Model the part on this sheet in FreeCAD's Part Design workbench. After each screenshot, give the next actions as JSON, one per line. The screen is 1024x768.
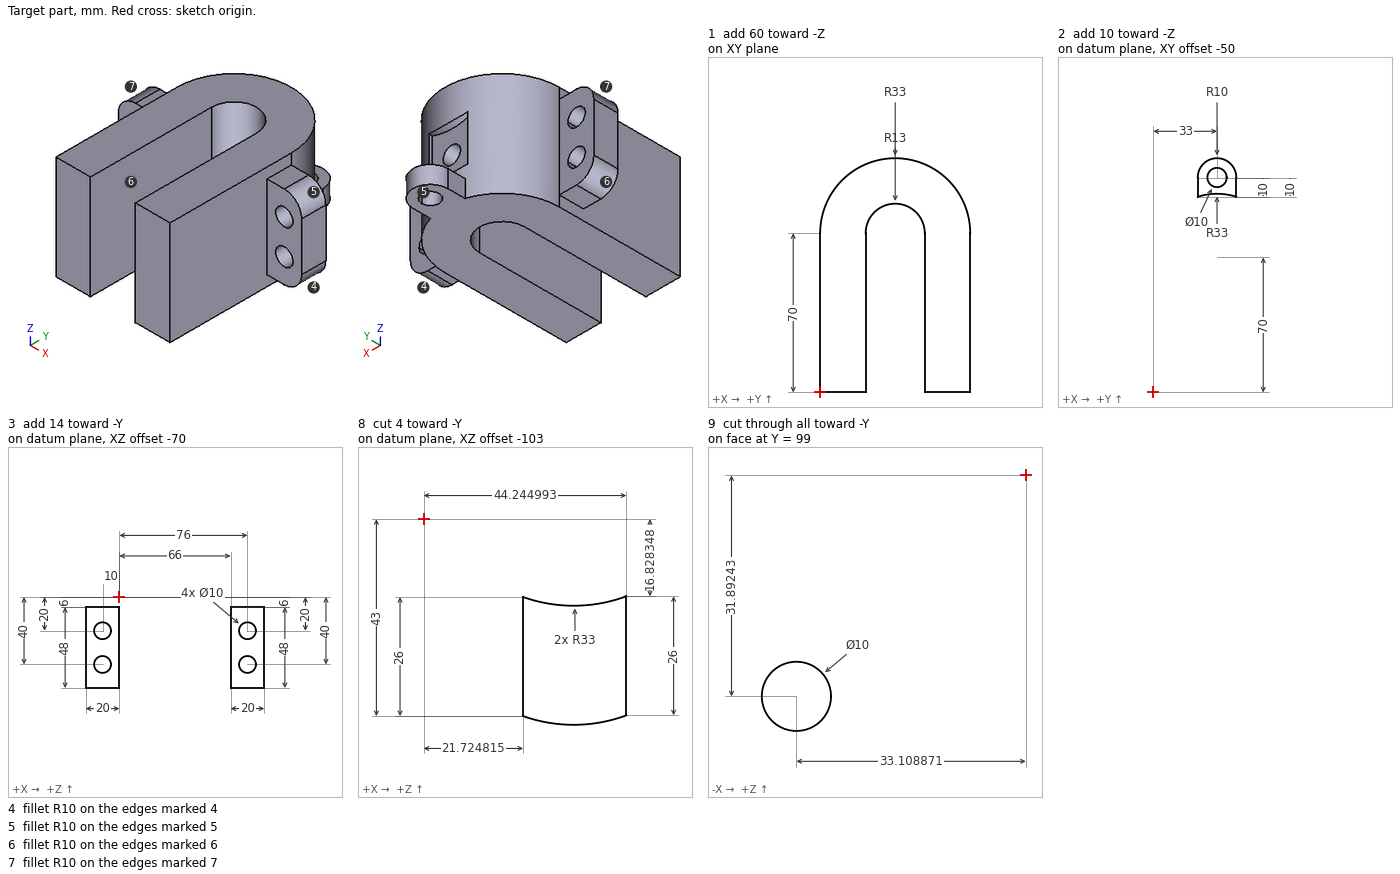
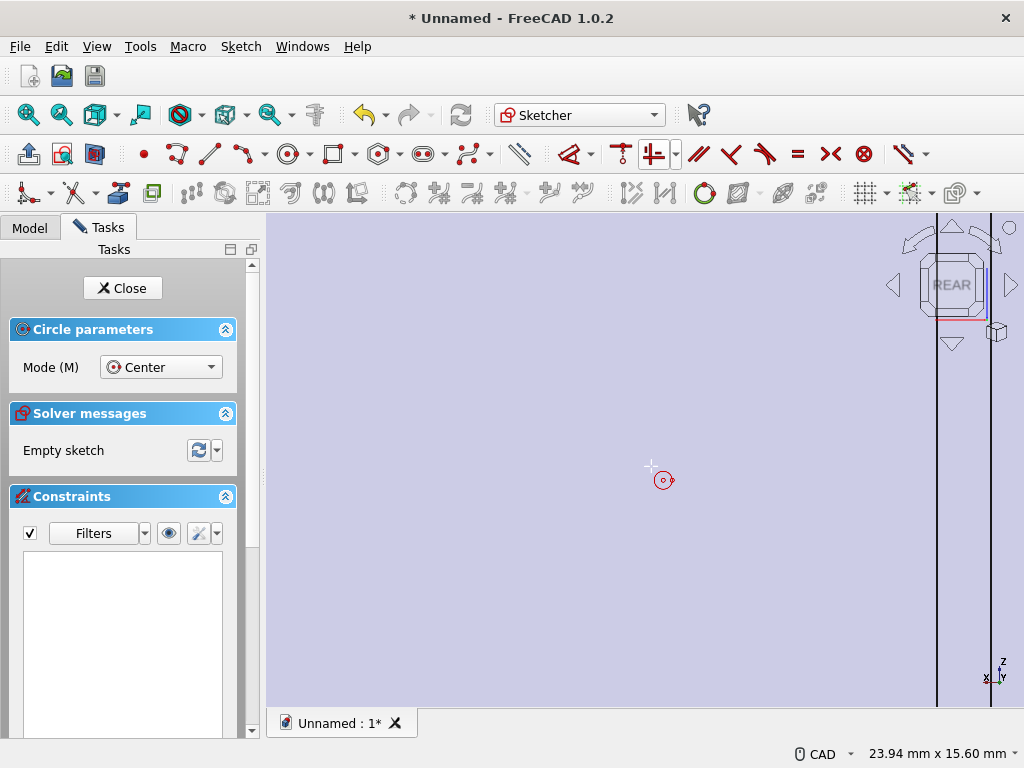
{"action": "left_click", "coordinate": [576, 455]}
{"action": "mouse_move", "coordinate": [688, 343]}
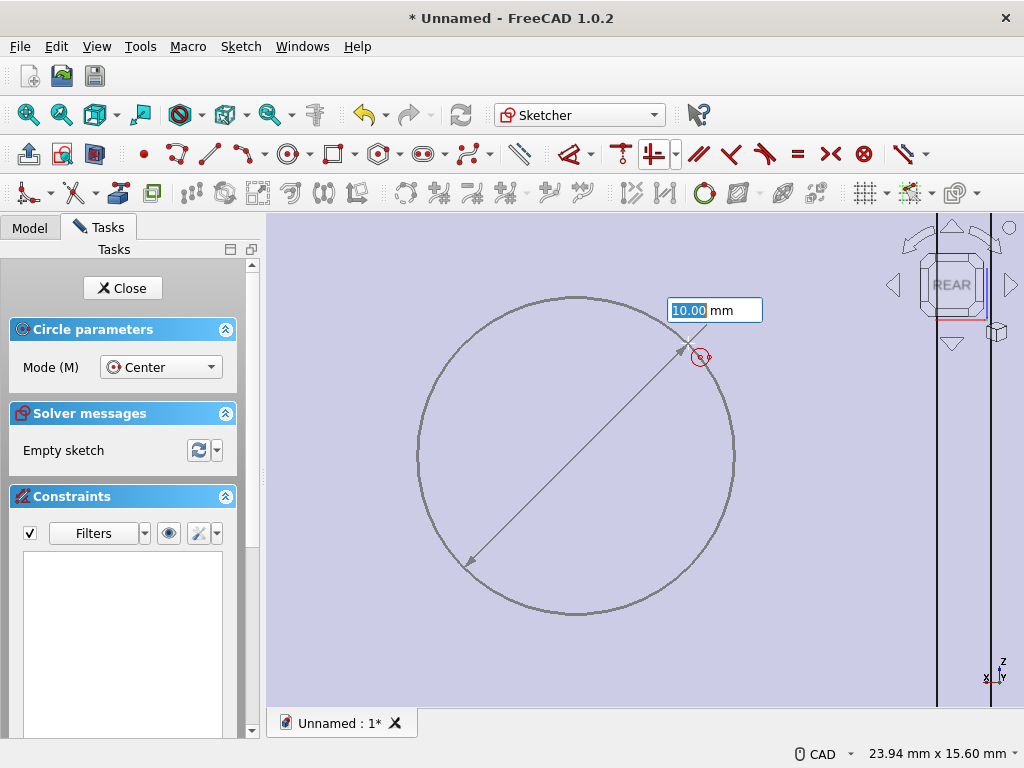
{"action": "type", "text": "10"}
{"action": "key", "text": "Return"}
{"action": "key", "text": "Escape"}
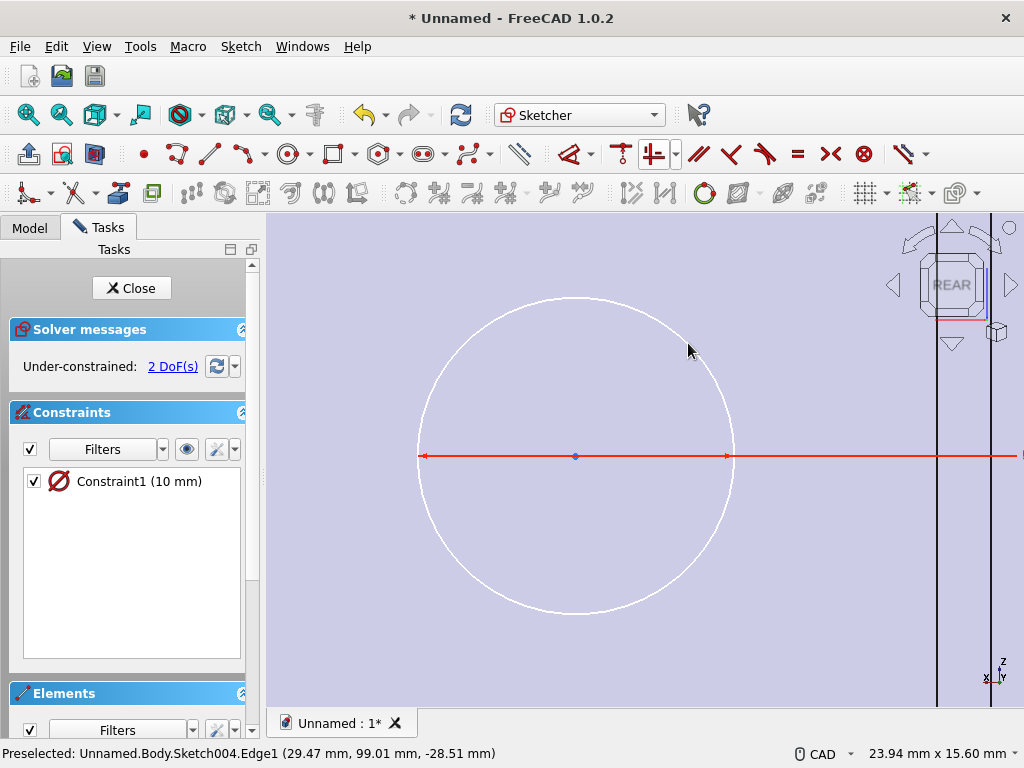
{"action": "left_click", "coordinate": [568, 154]}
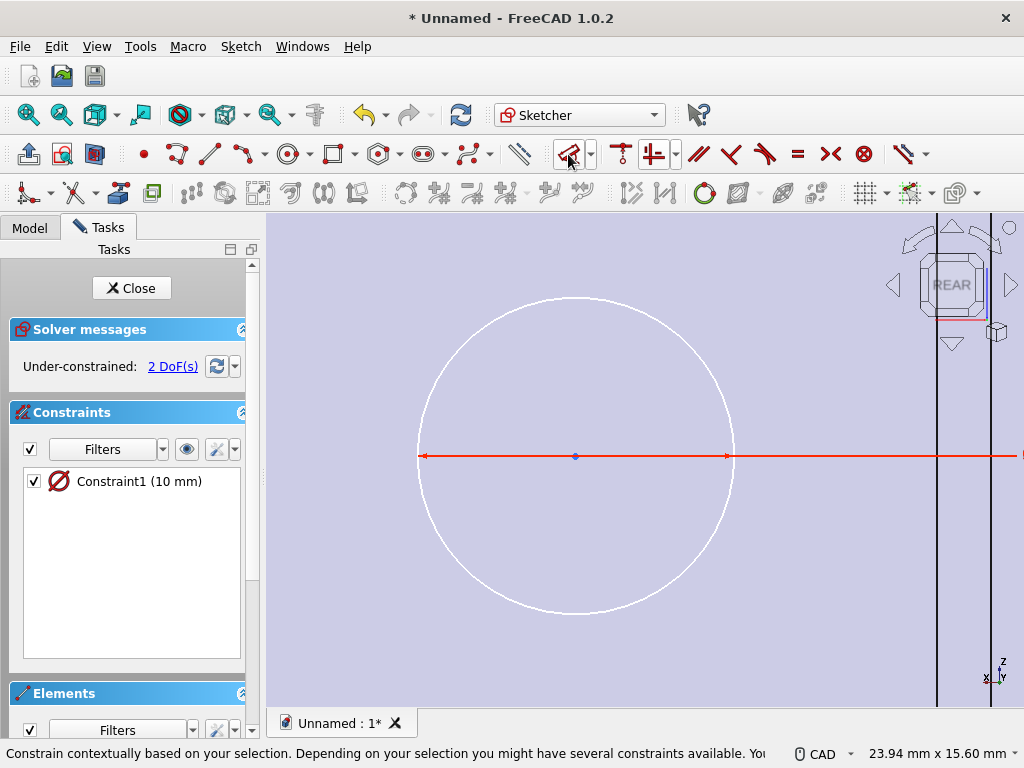
{"action": "left_click", "coordinate": [576, 456]}
{"action": "left_click", "coordinate": [542, 348]}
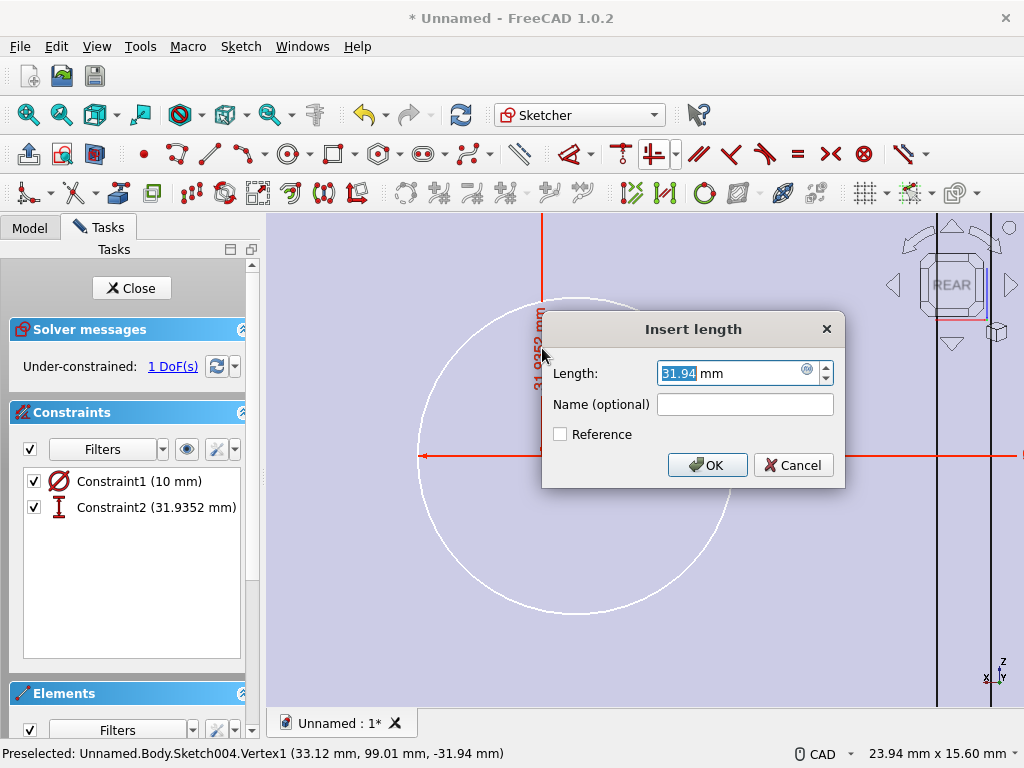
{"action": "type", "text": "31.89243"}
{"action": "key", "text": "Return"}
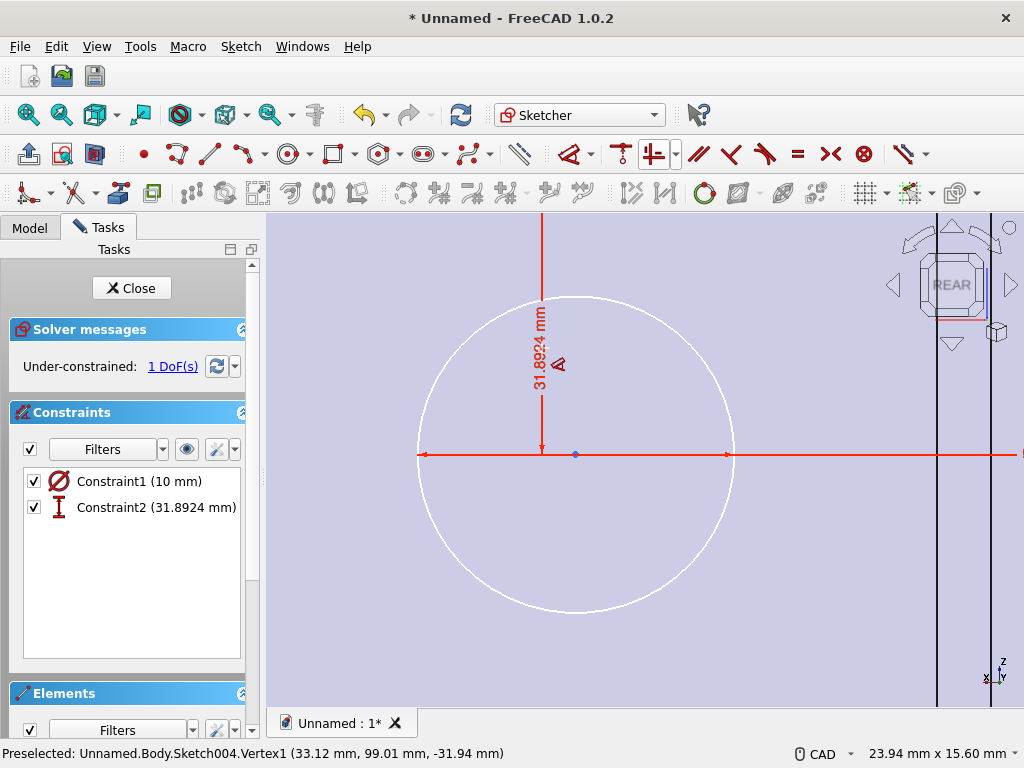
{"action": "left_click", "coordinate": [576, 455]}
{"action": "left_click", "coordinate": [652, 489]}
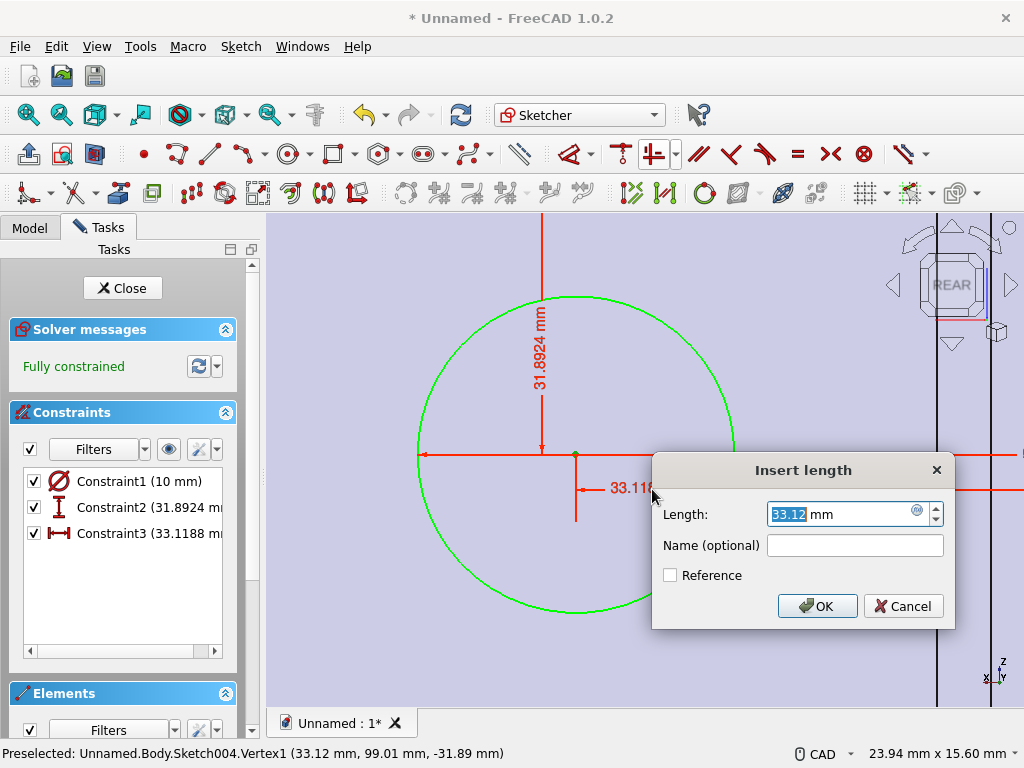
{"action": "type", "text": "33.108871"}
{"action": "key", "text": "Return"}
{"action": "key", "text": "Escape"}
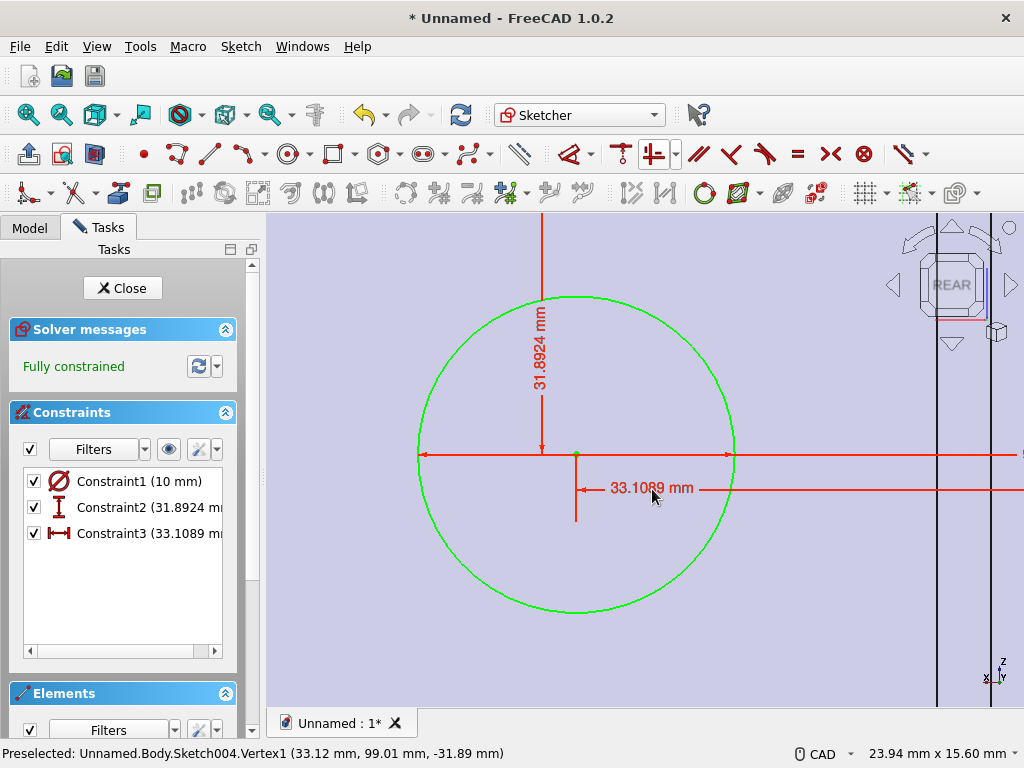
{"action": "left_click", "coordinate": [123, 288]}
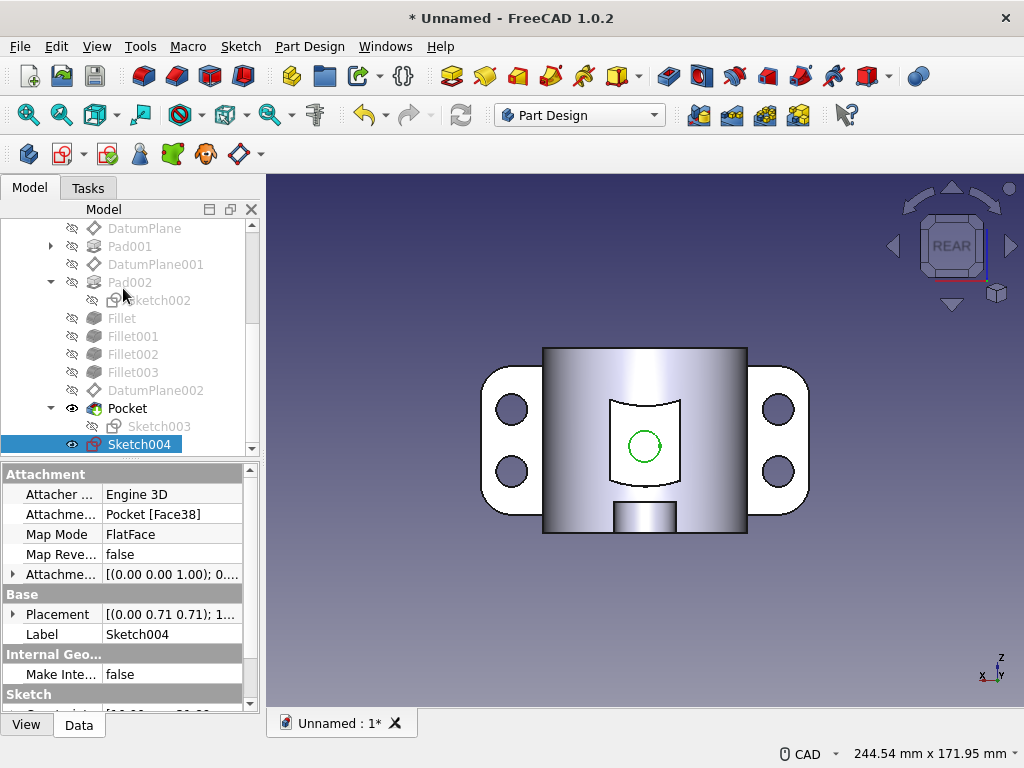
{"action": "left_click", "coordinate": [669, 76]}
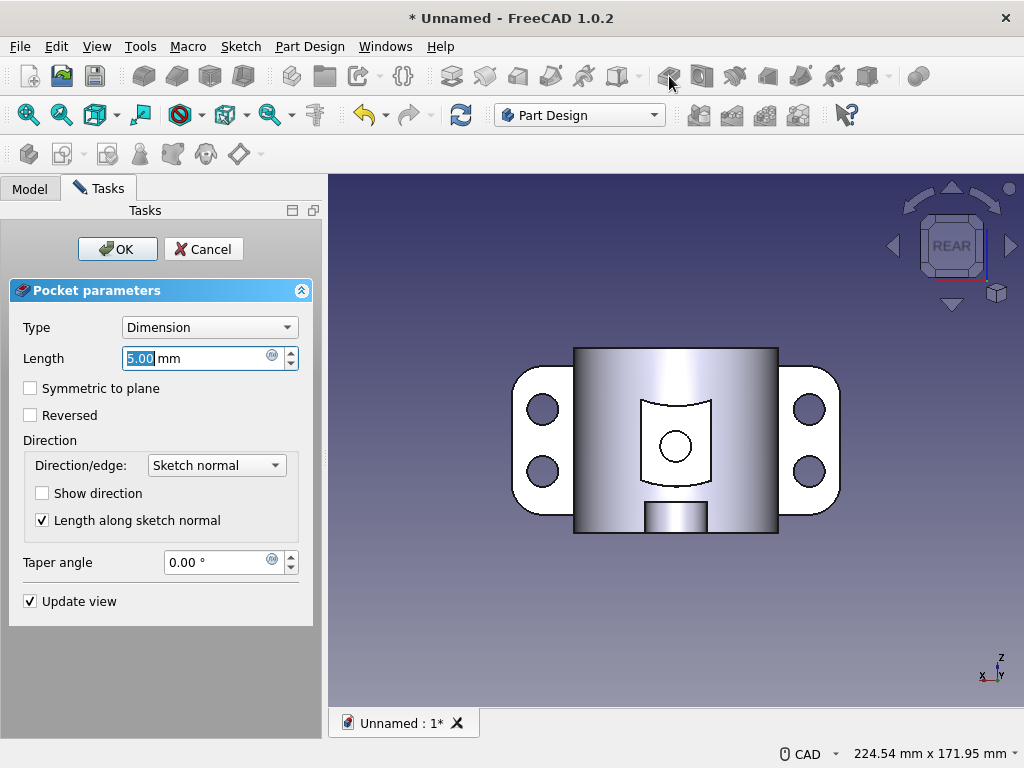
{"action": "left_click", "coordinate": [210, 328]}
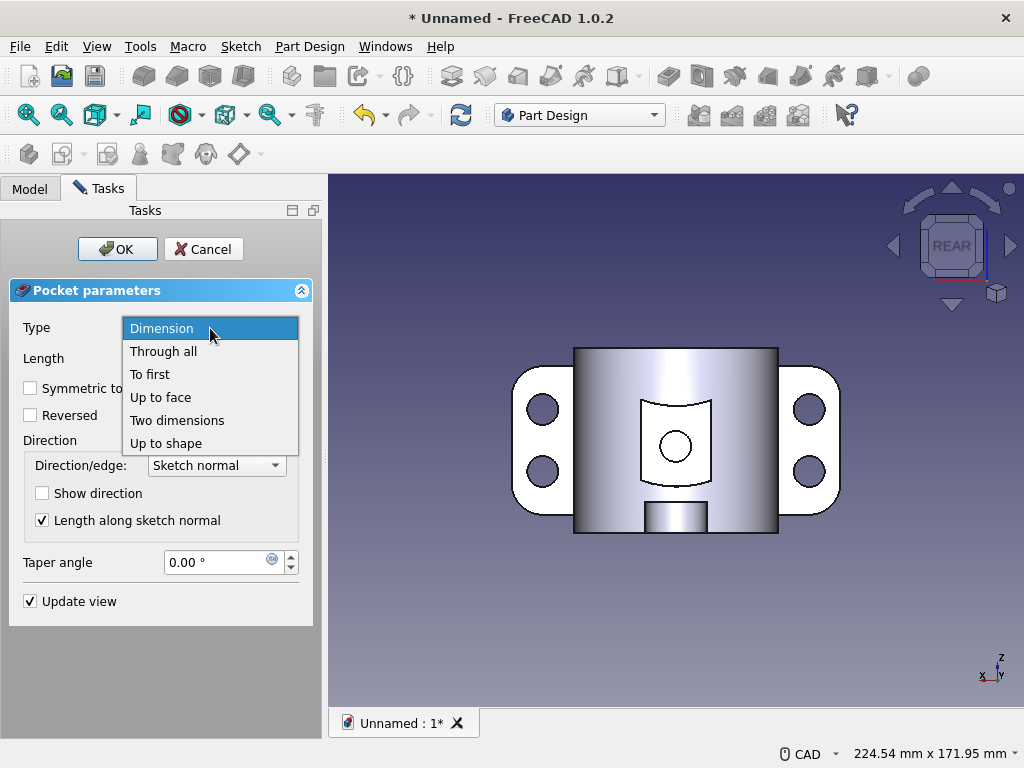
{"action": "left_click", "coordinate": [208, 352]}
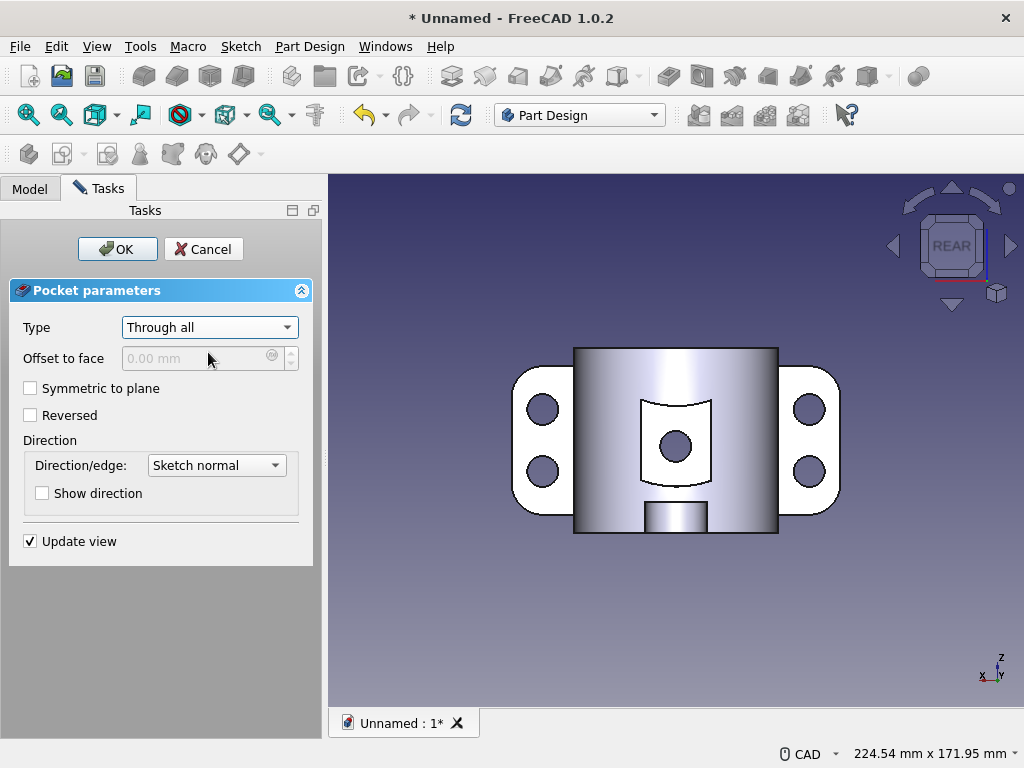
{"action": "left_click", "coordinate": [118, 249]}